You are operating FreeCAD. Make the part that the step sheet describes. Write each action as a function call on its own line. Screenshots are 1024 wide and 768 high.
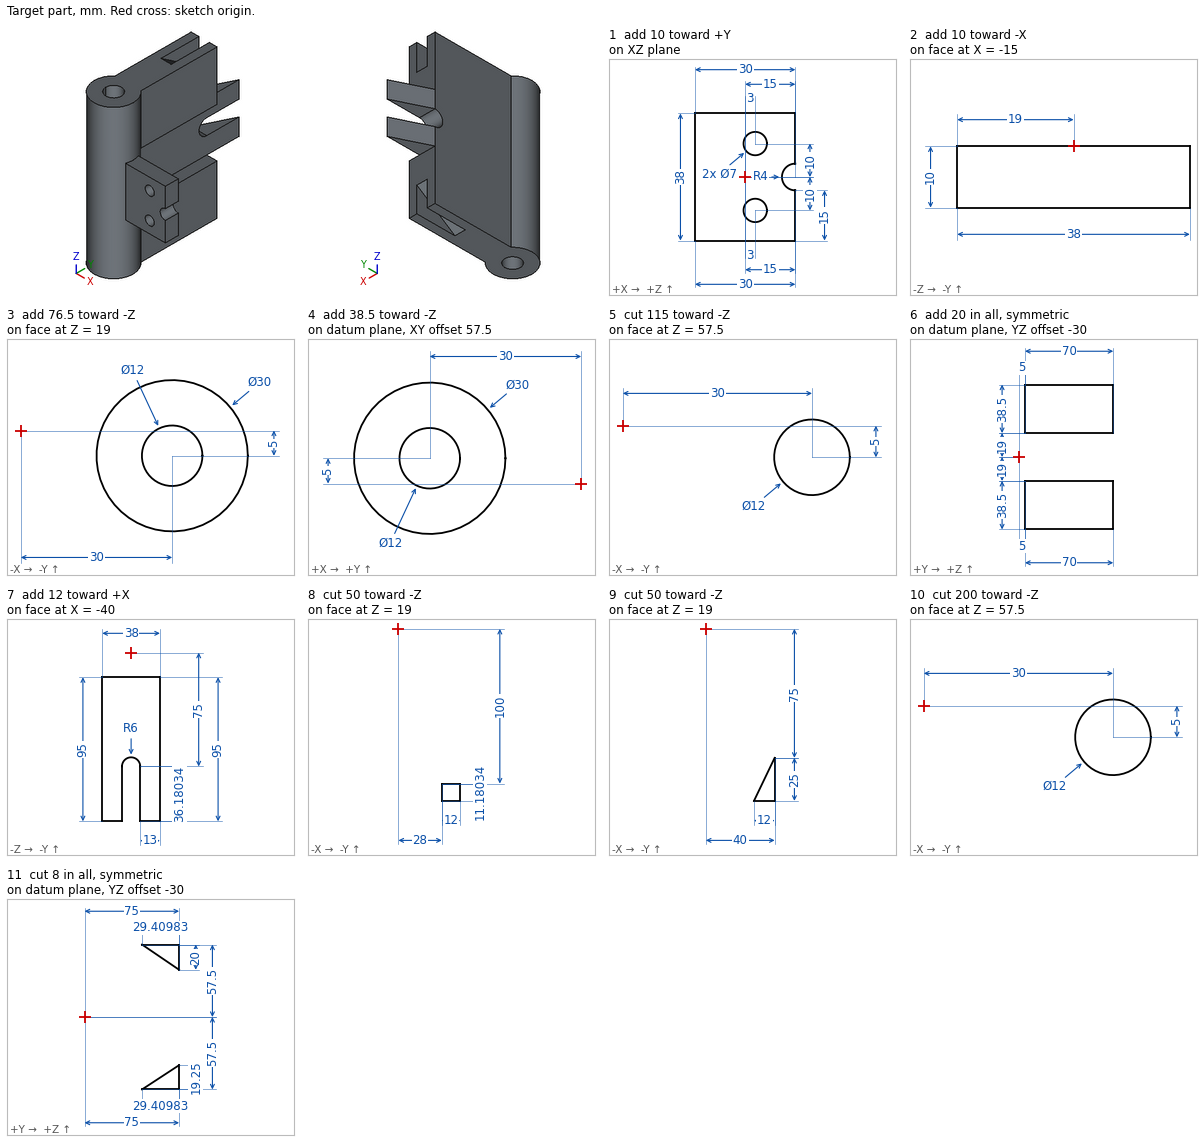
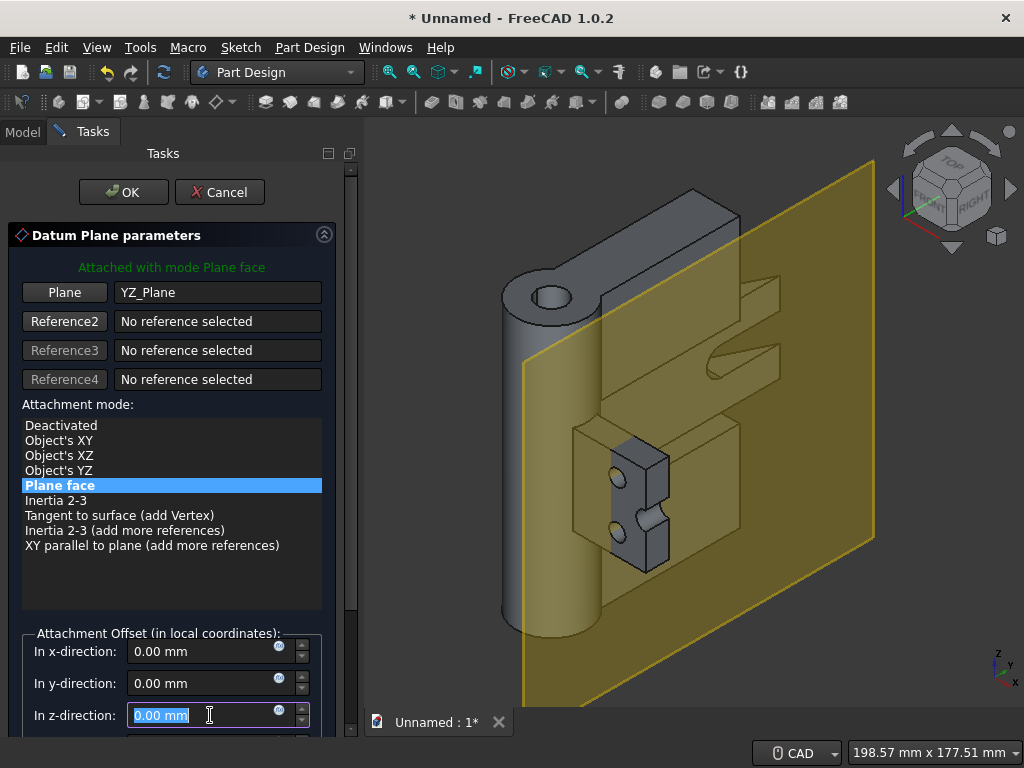
text(-30)
key(Tab)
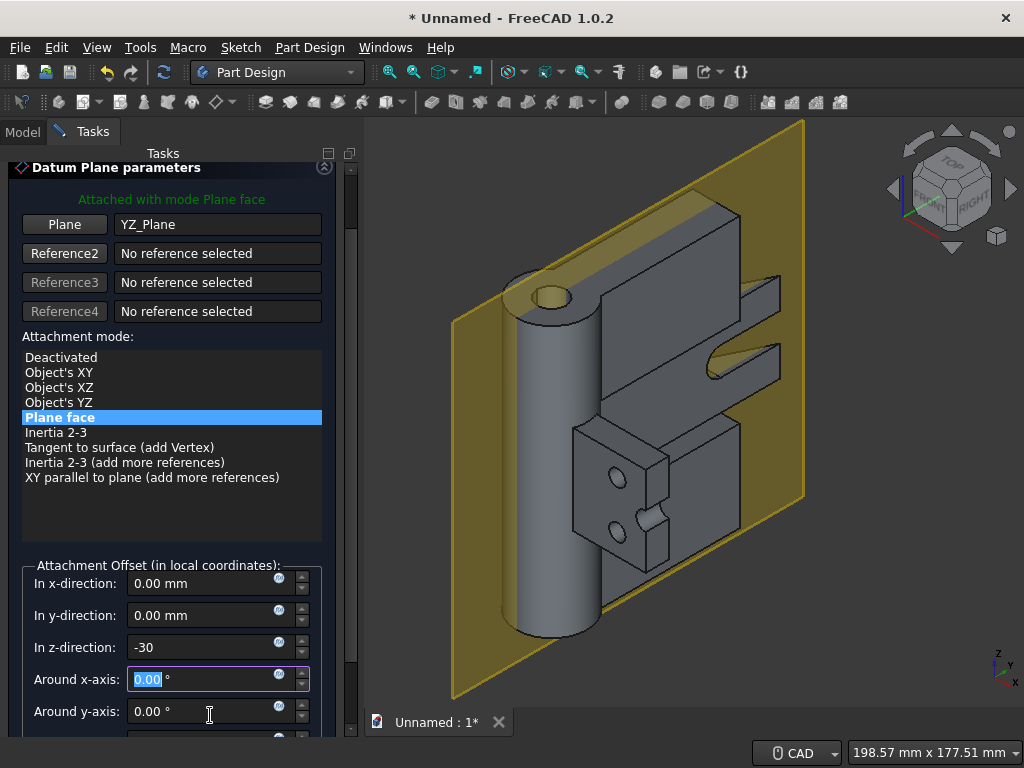
scroll(351, 450, up, 2)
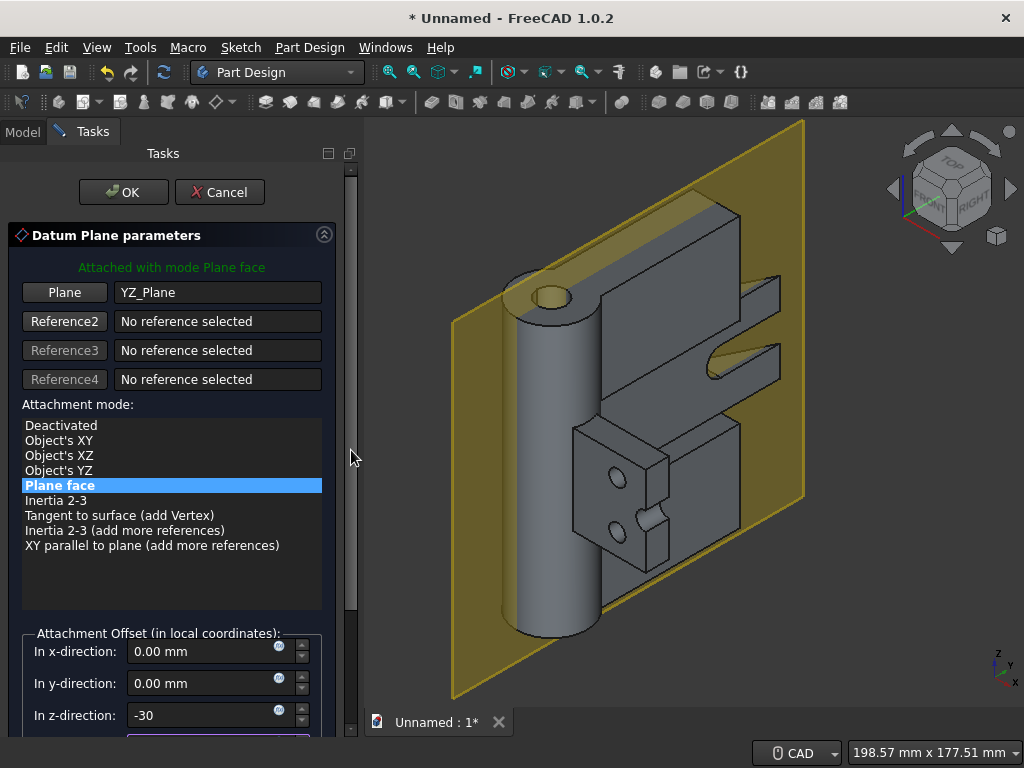
click(124, 192)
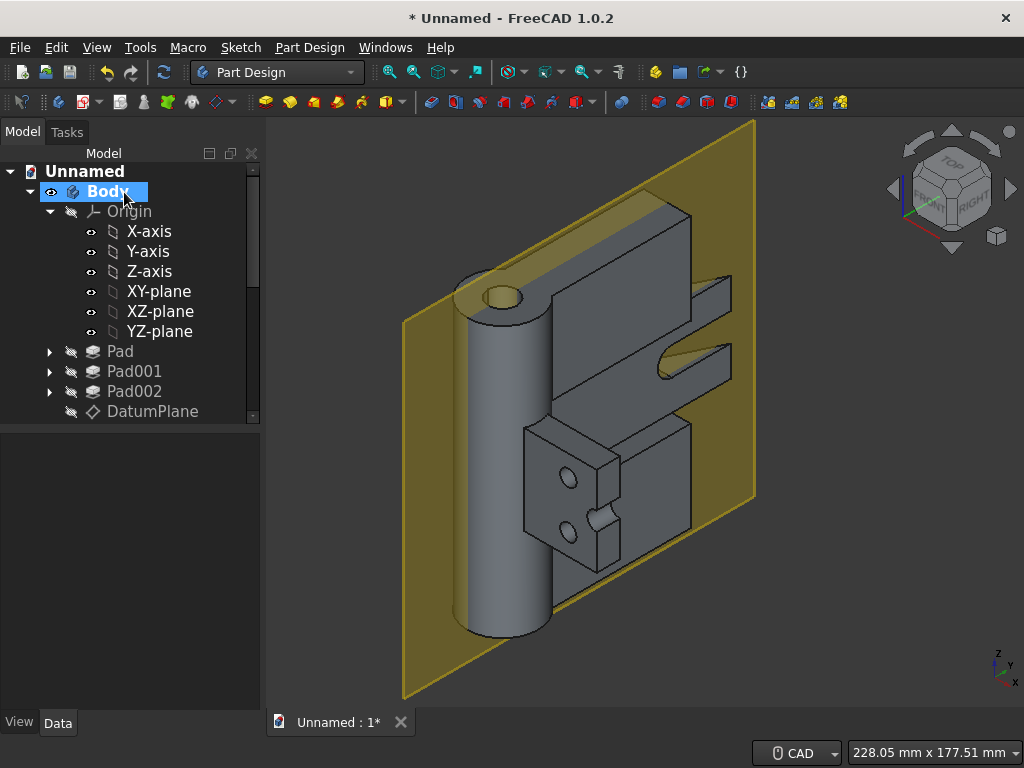
scroll(100, 287, down, 3)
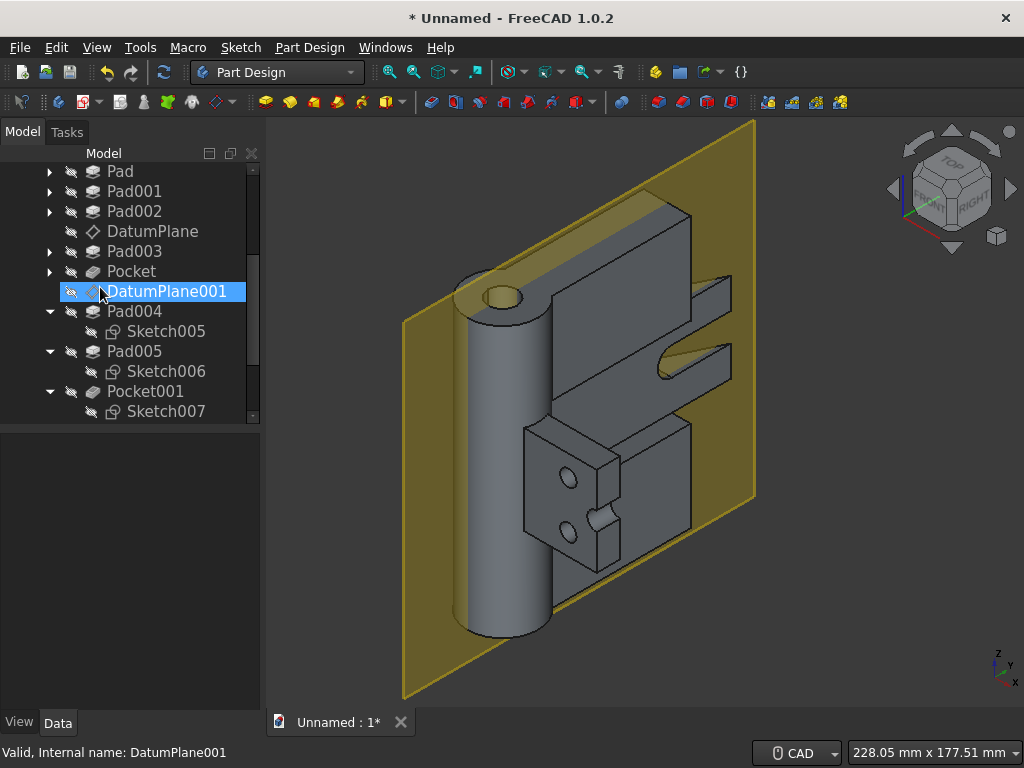
scroll(140, 287, up, 15)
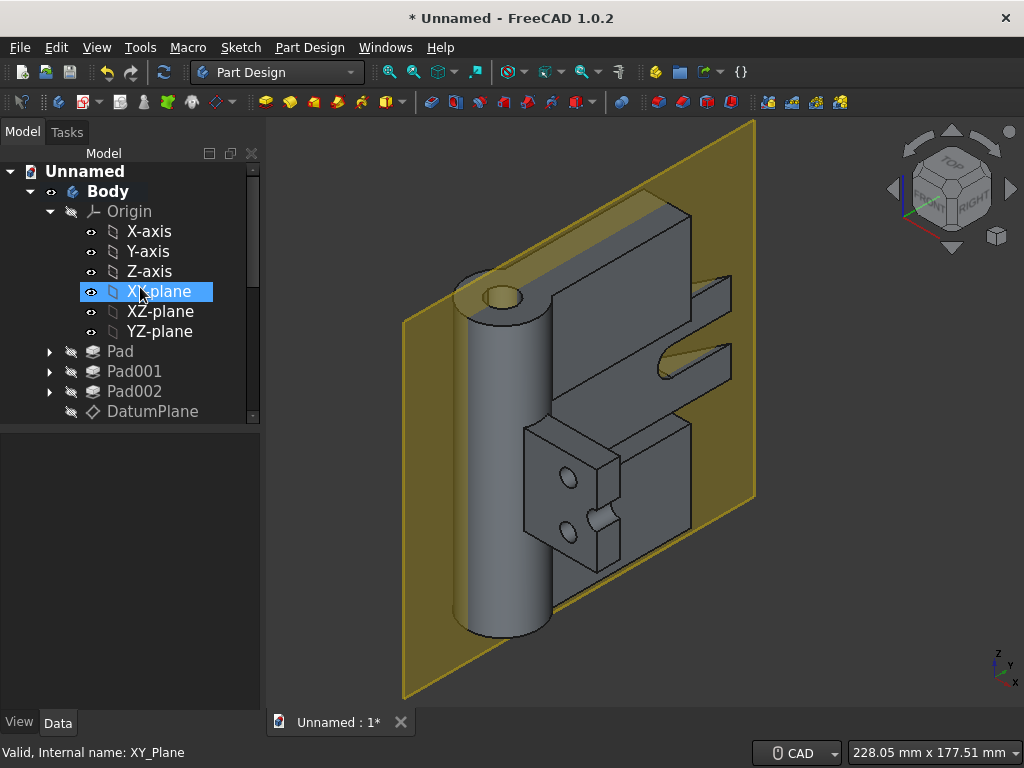
scroll(100, 287, down, 6)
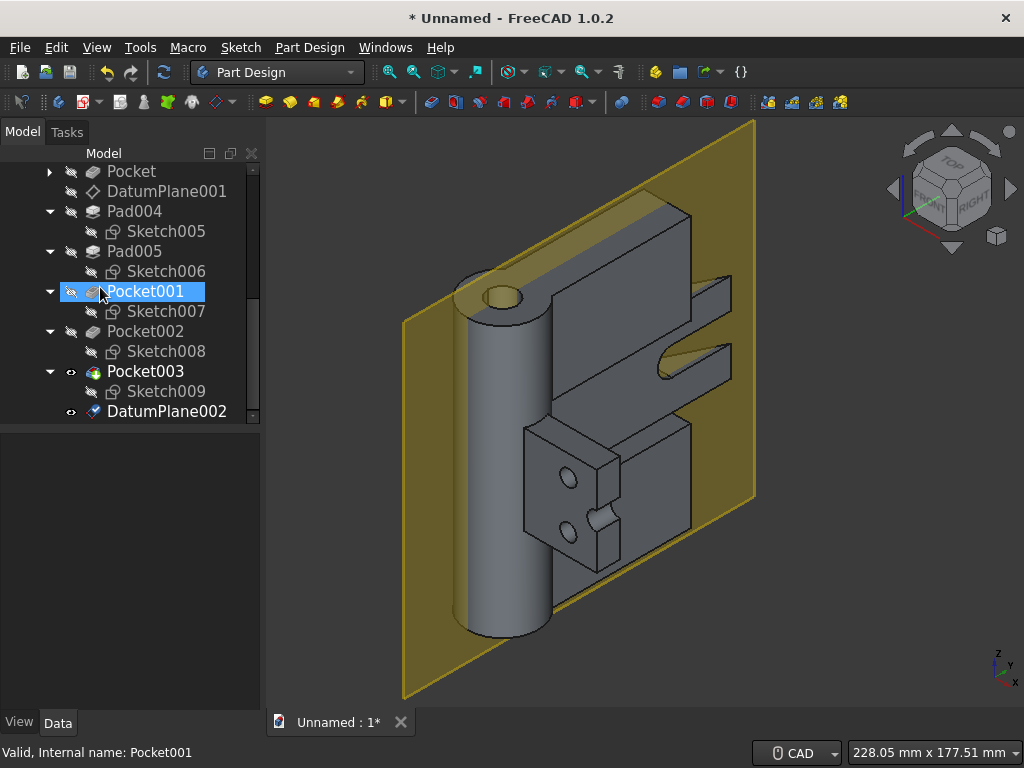
click(116, 412)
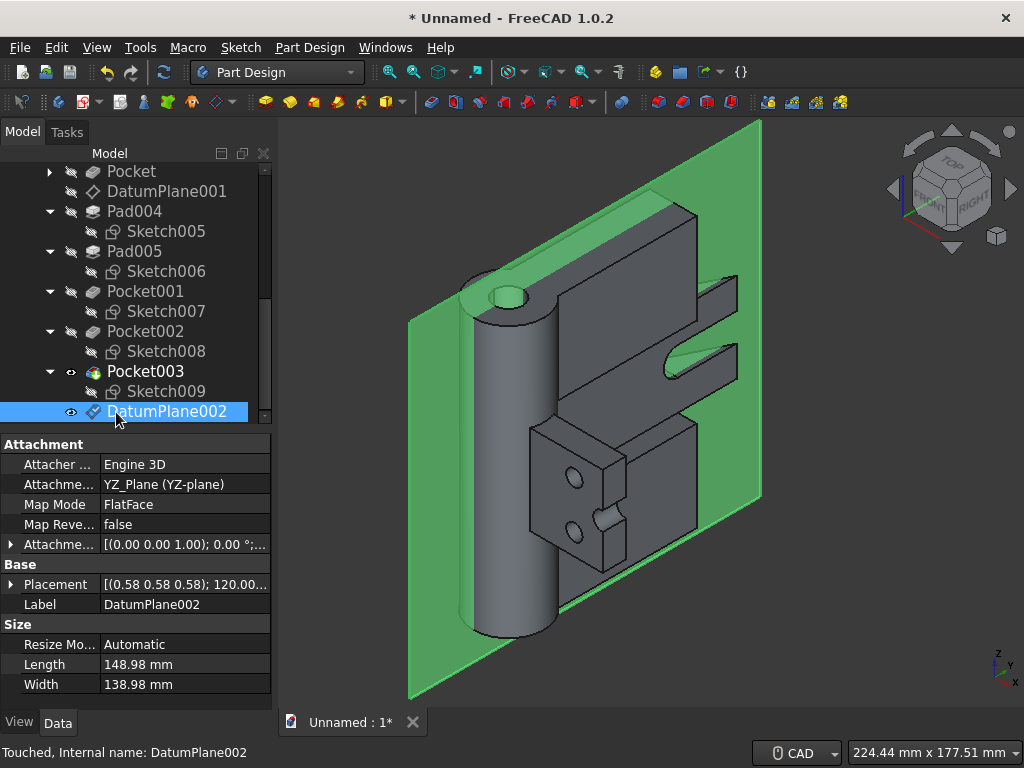
click(84, 102)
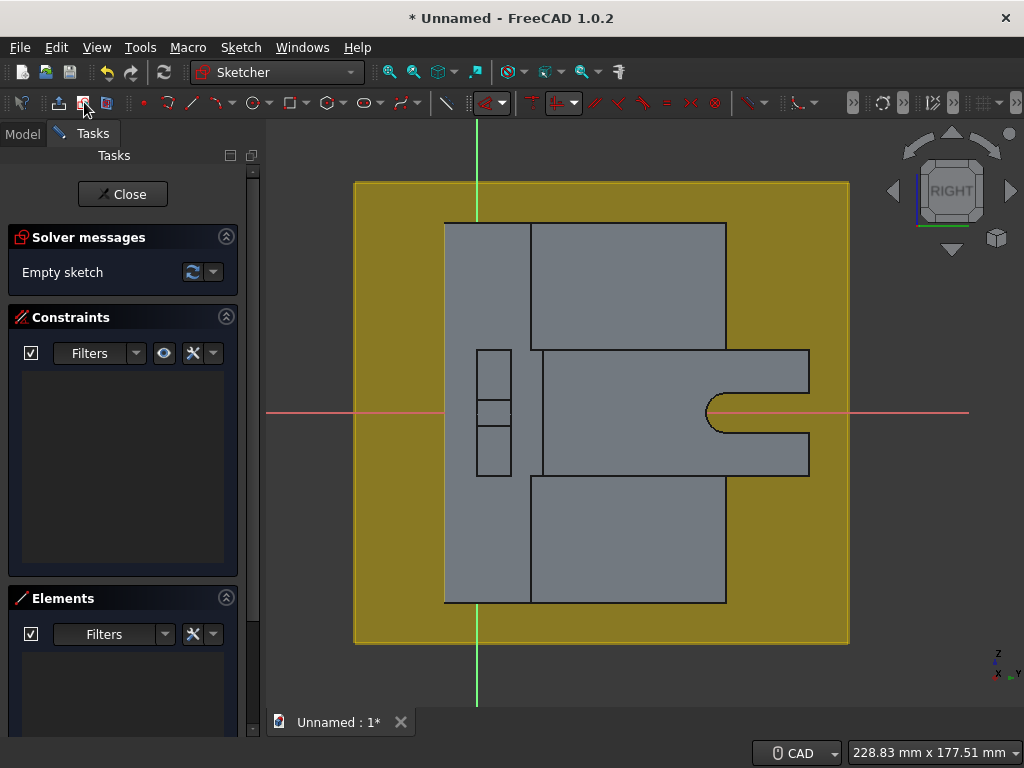
click(108, 104)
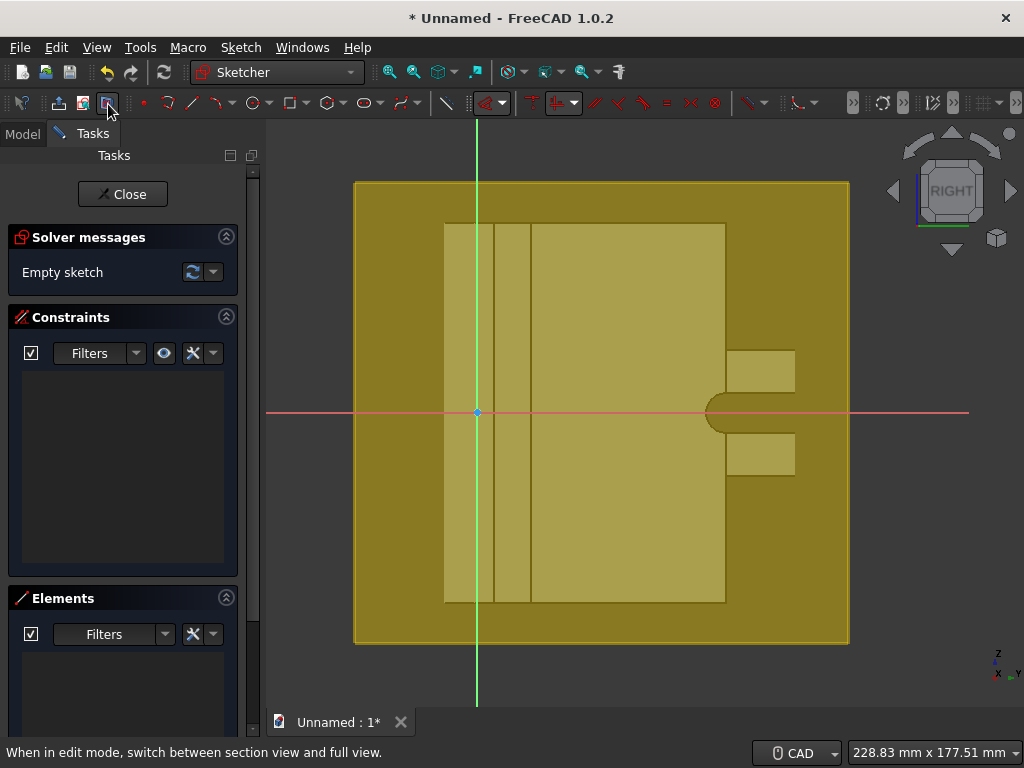
click(168, 104)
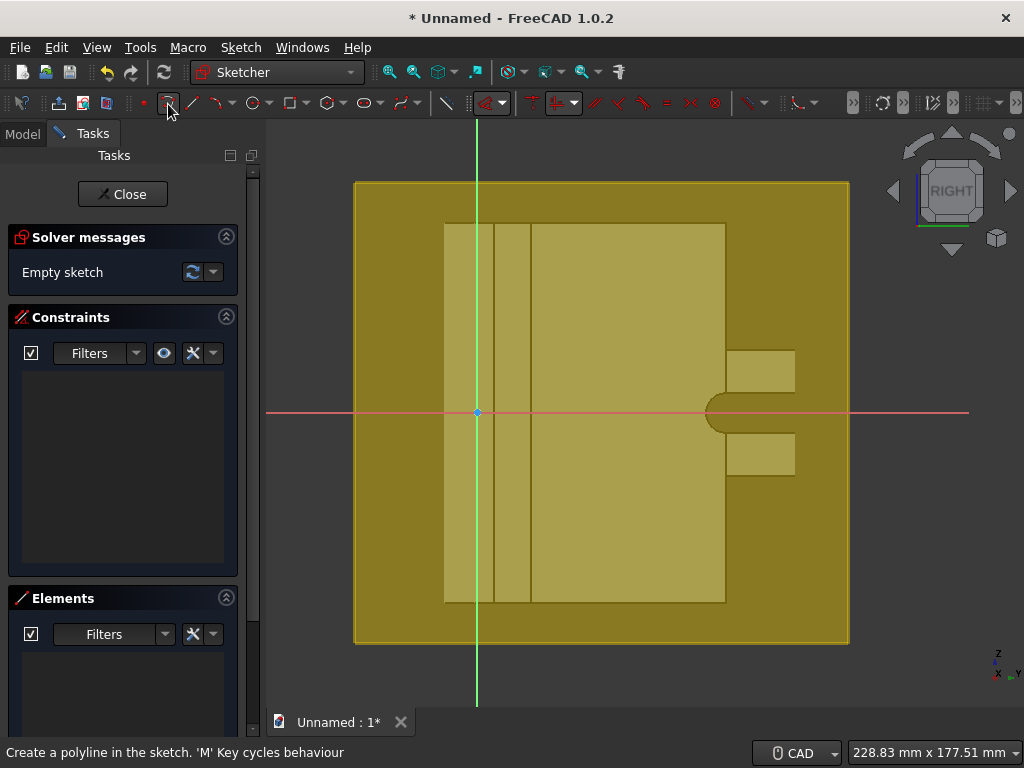
click(628, 603)
click(726, 603)
click(726, 540)
click(628, 604)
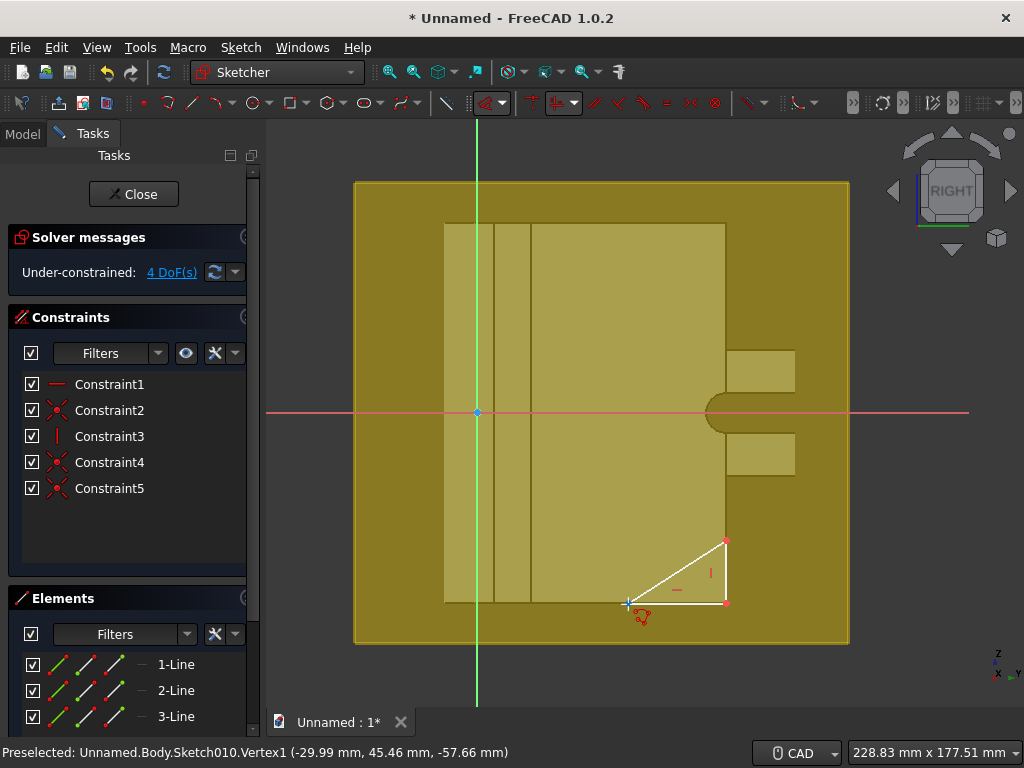
click(628, 223)
click(726, 289)
click(726, 223)
click(628, 224)
key(Escape)
key(Escape)